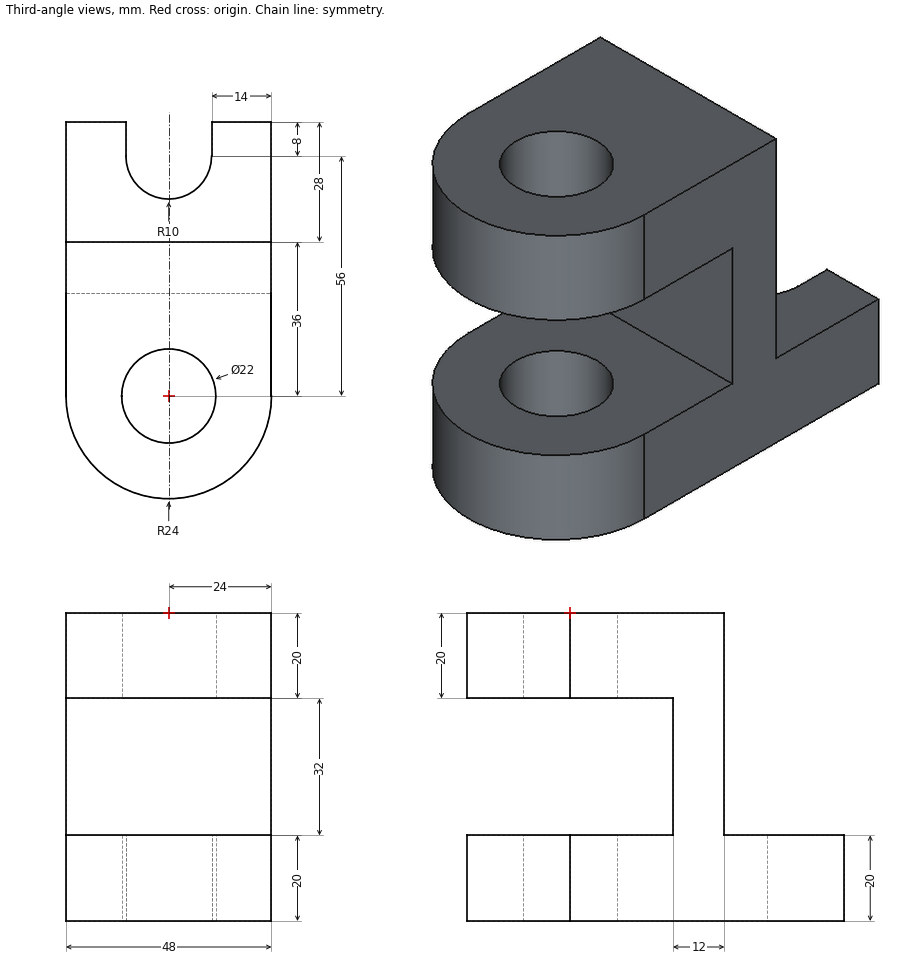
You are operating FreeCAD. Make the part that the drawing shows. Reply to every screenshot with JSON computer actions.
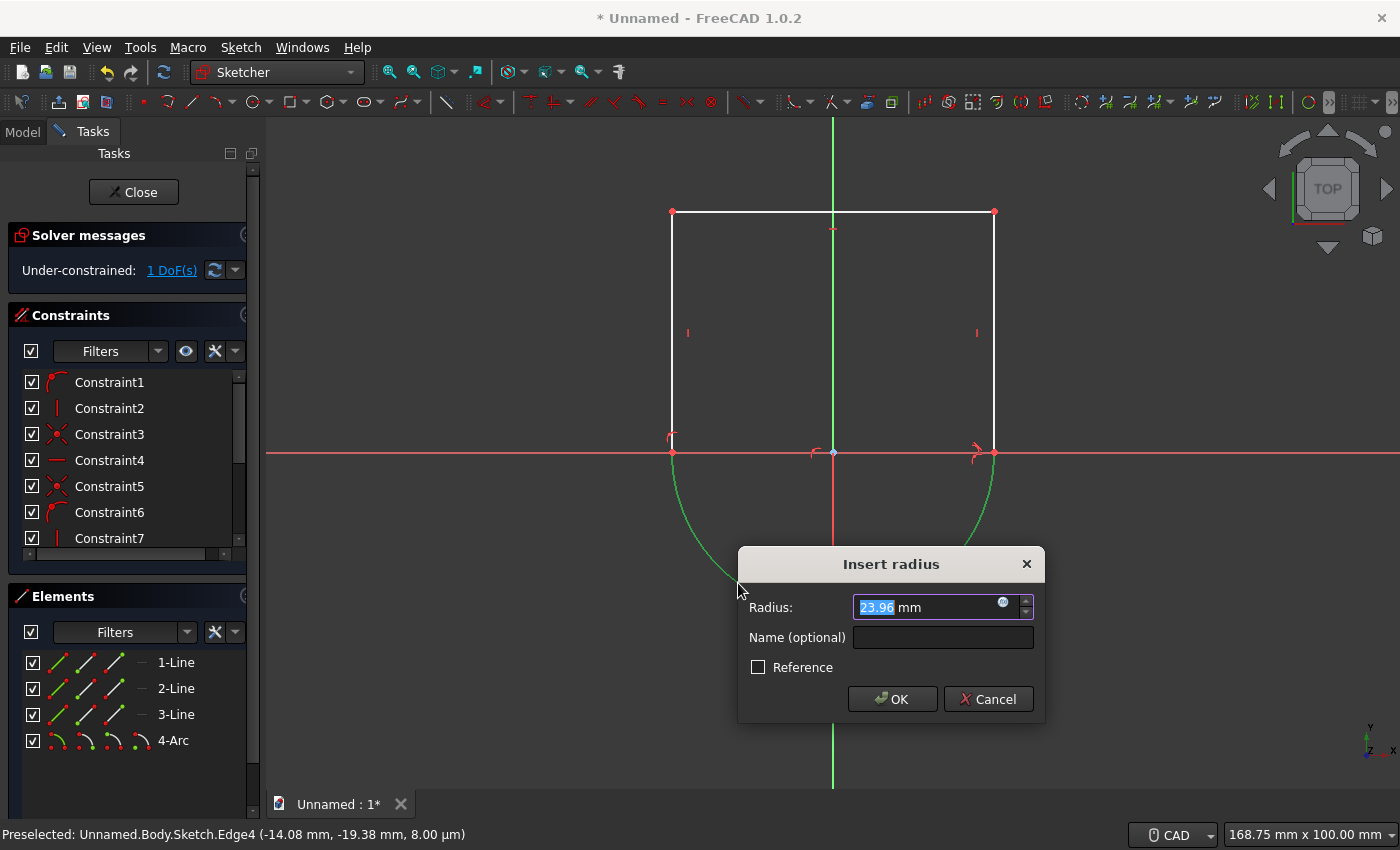
{"action": "type", "text": "24"}
{"action": "key", "text": "Return"}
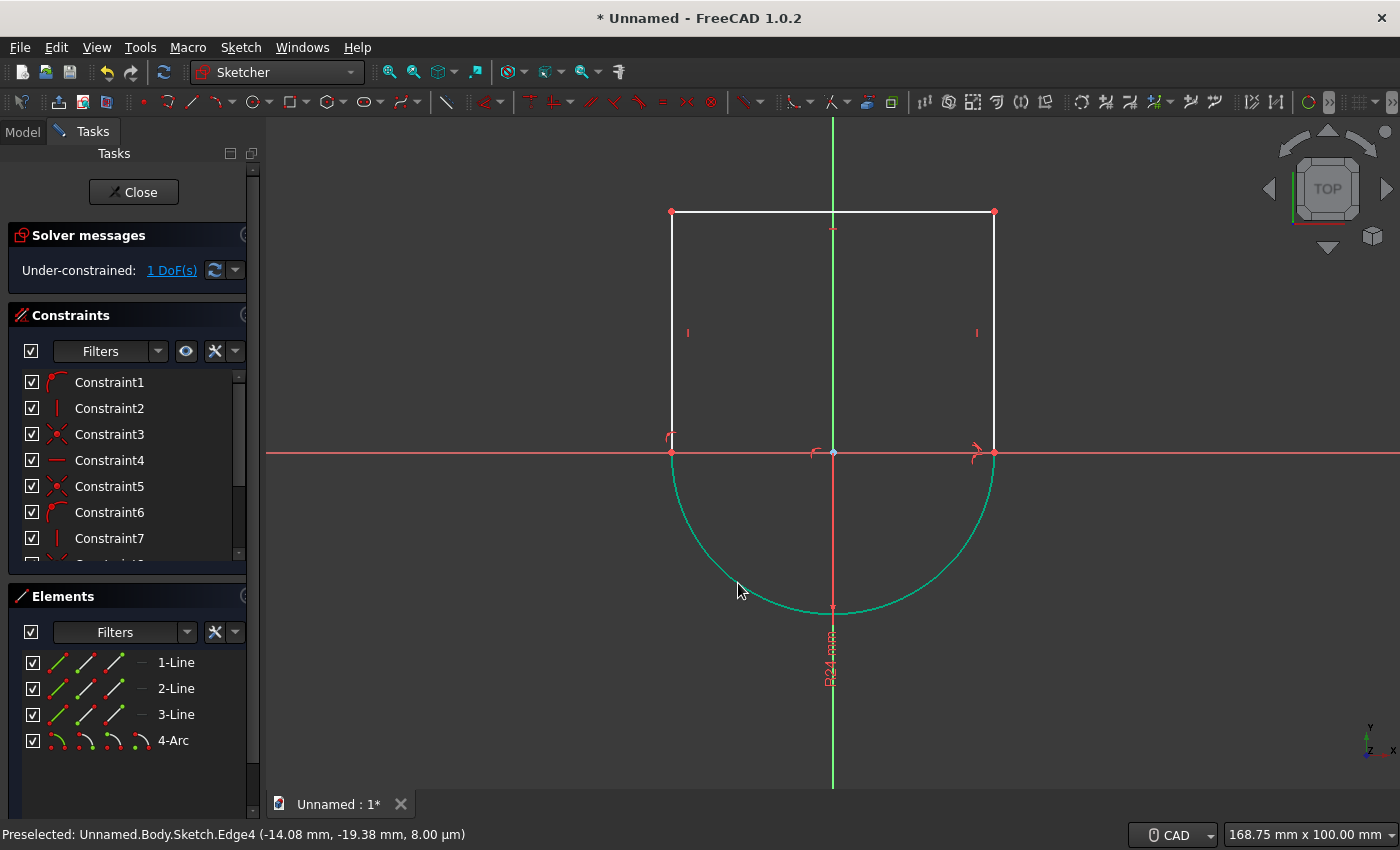
{"action": "left_click", "coordinate": [994, 381]}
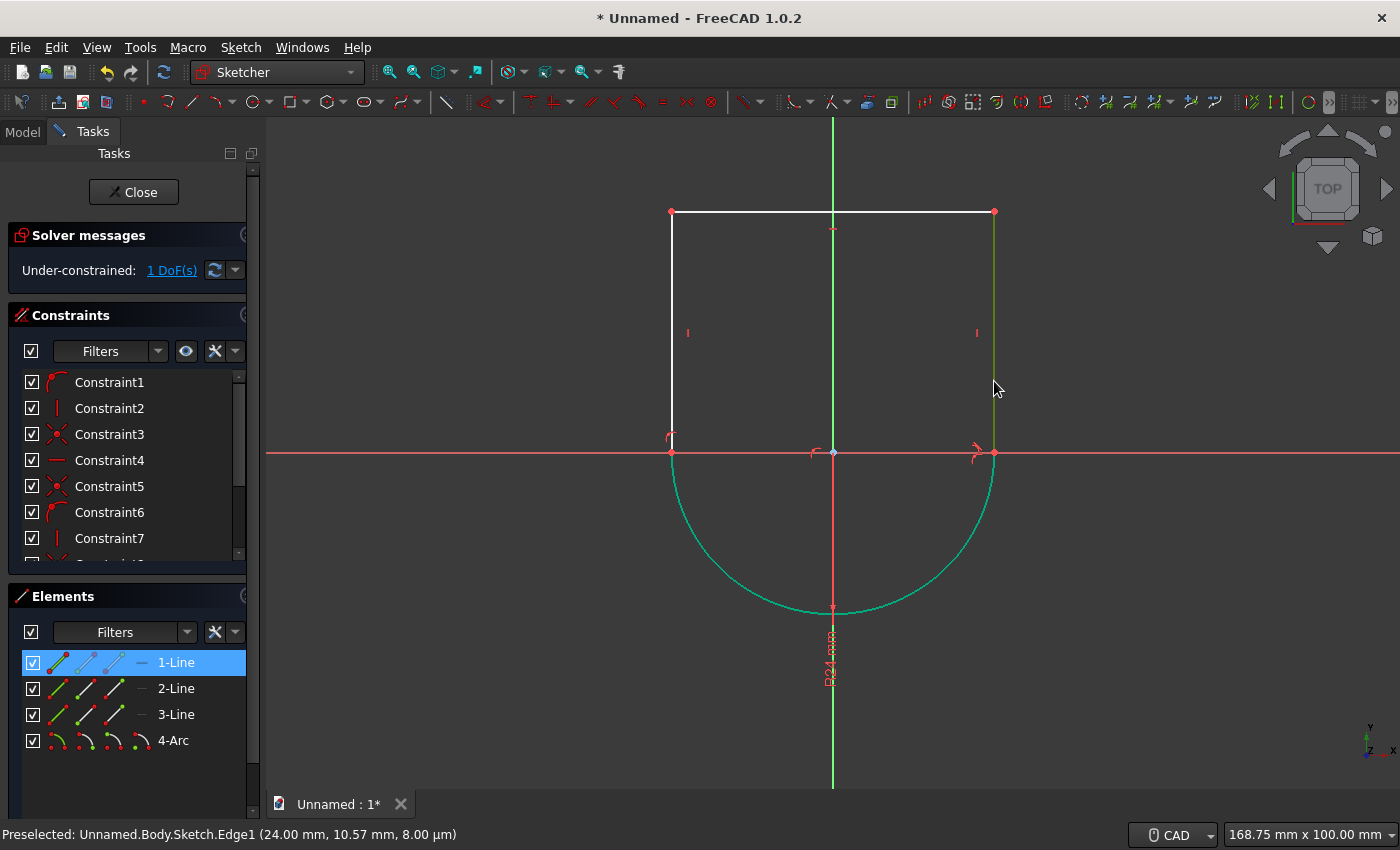
{"action": "left_click", "coordinate": [502, 102]}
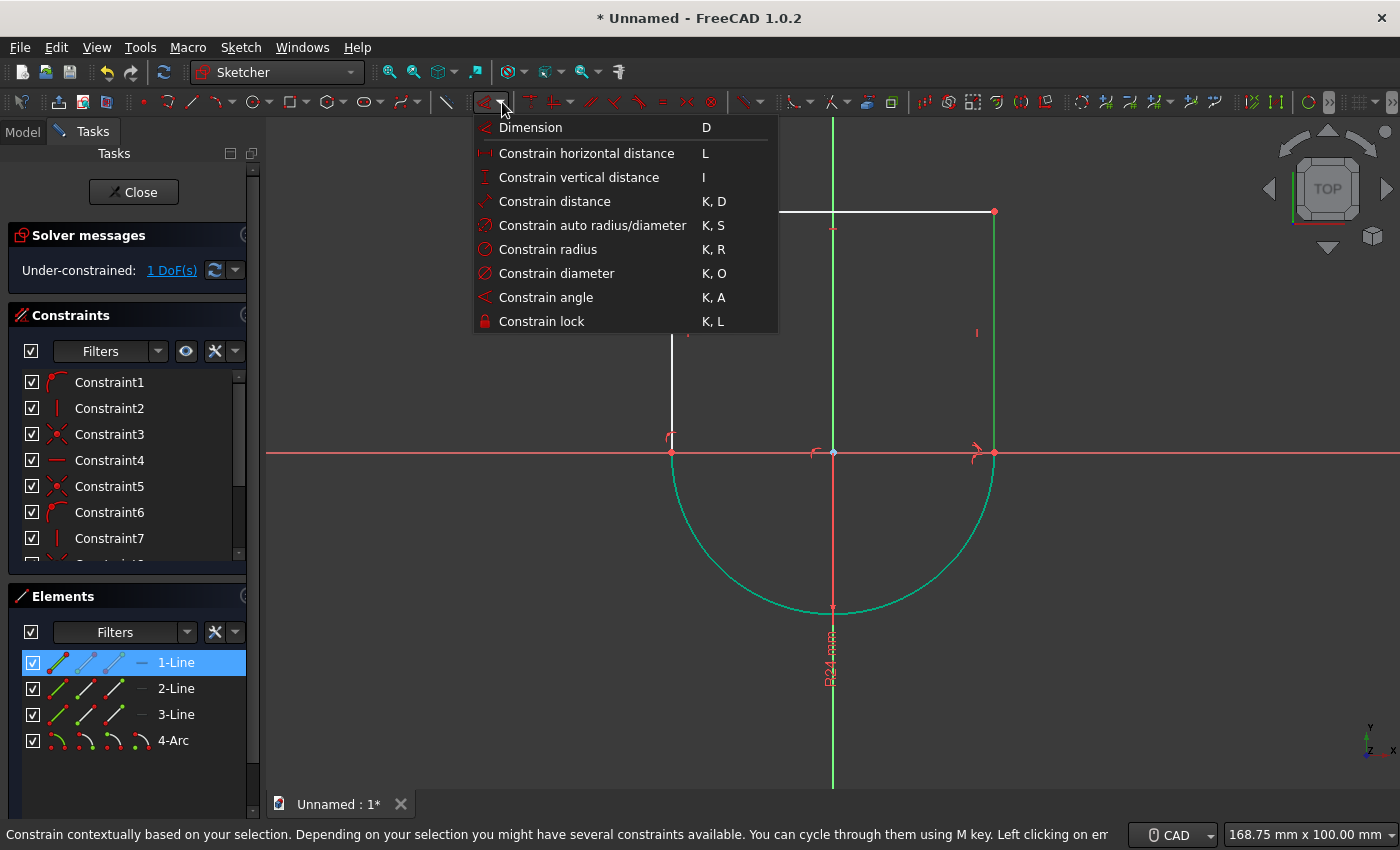
{"action": "left_click", "coordinate": [626, 177]}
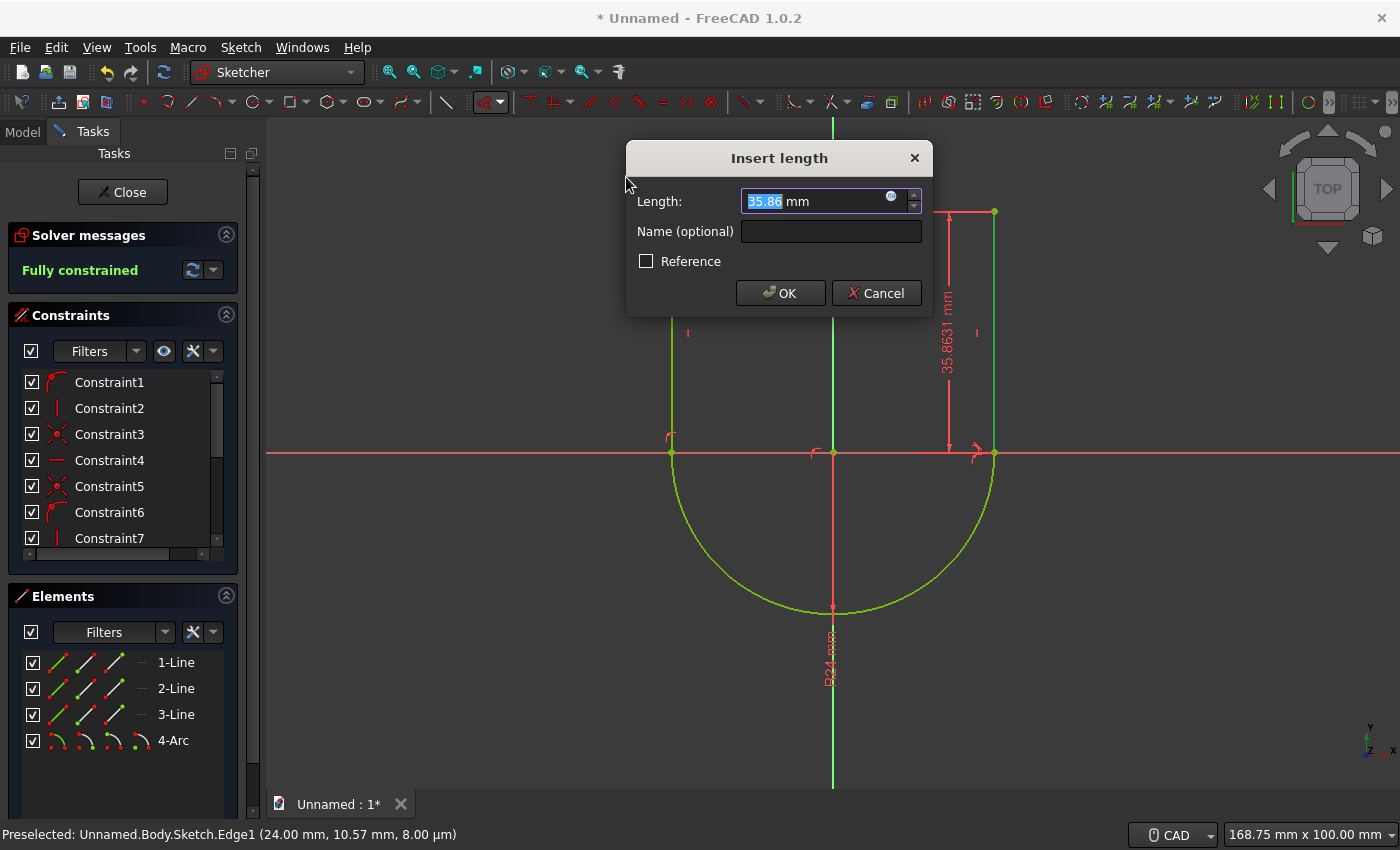
{"action": "type", "text": "36"}
{"action": "key", "text": "Return"}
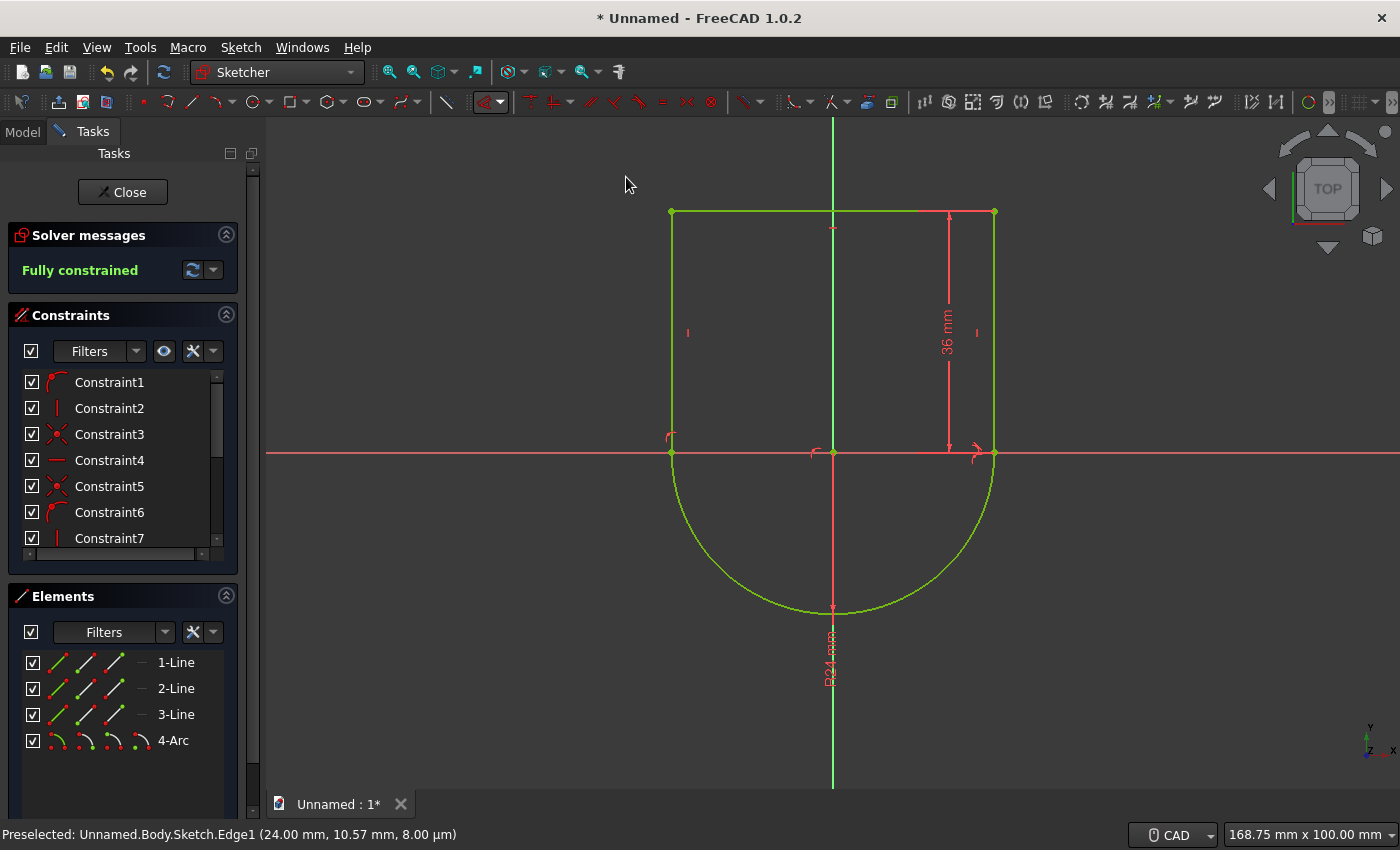
{"action": "left_click", "coordinate": [123, 192]}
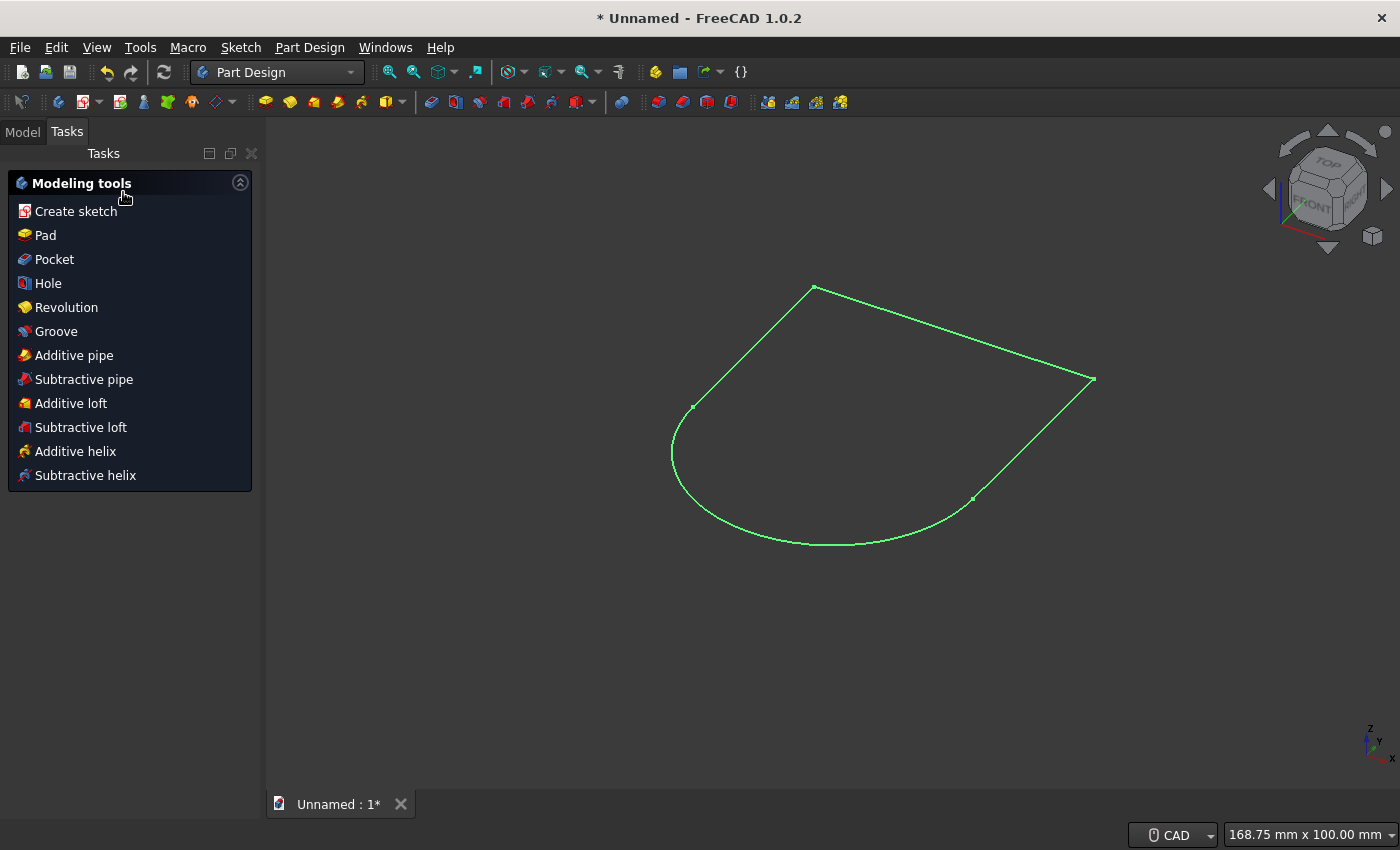
{"action": "left_click", "coordinate": [266, 102]}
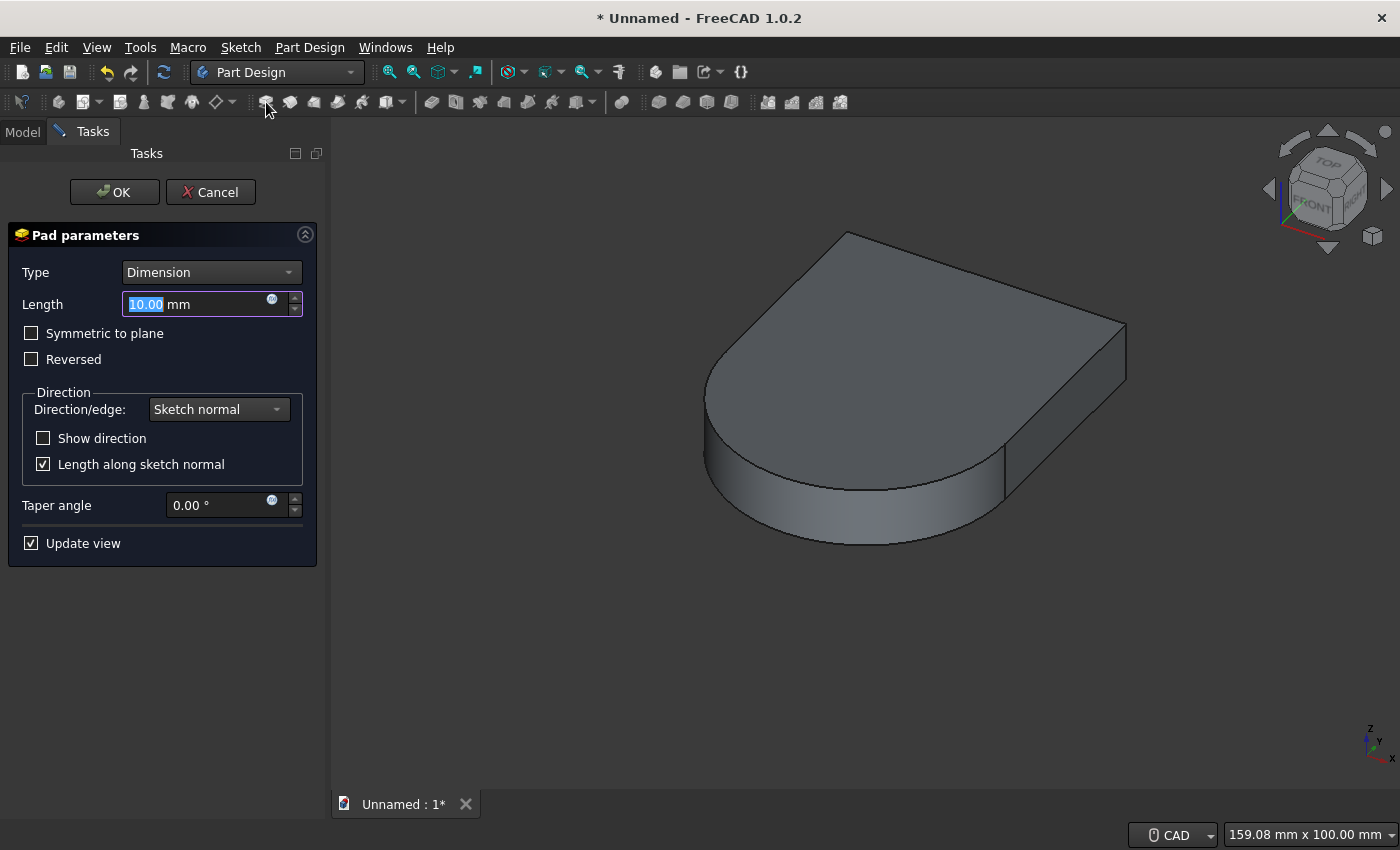
{"action": "type", "text": "20"}
{"action": "key", "text": "Tab"}